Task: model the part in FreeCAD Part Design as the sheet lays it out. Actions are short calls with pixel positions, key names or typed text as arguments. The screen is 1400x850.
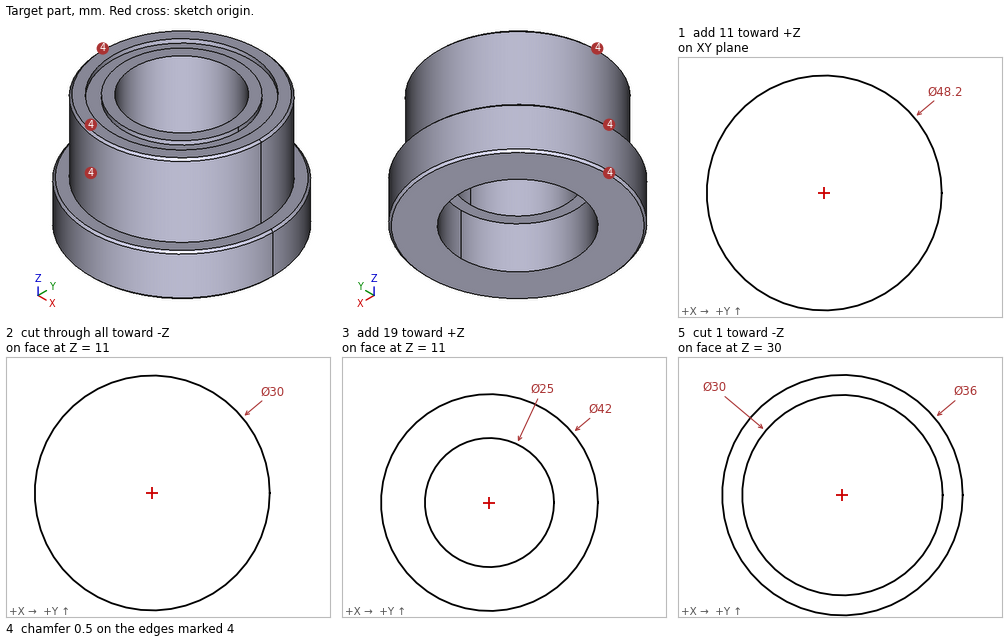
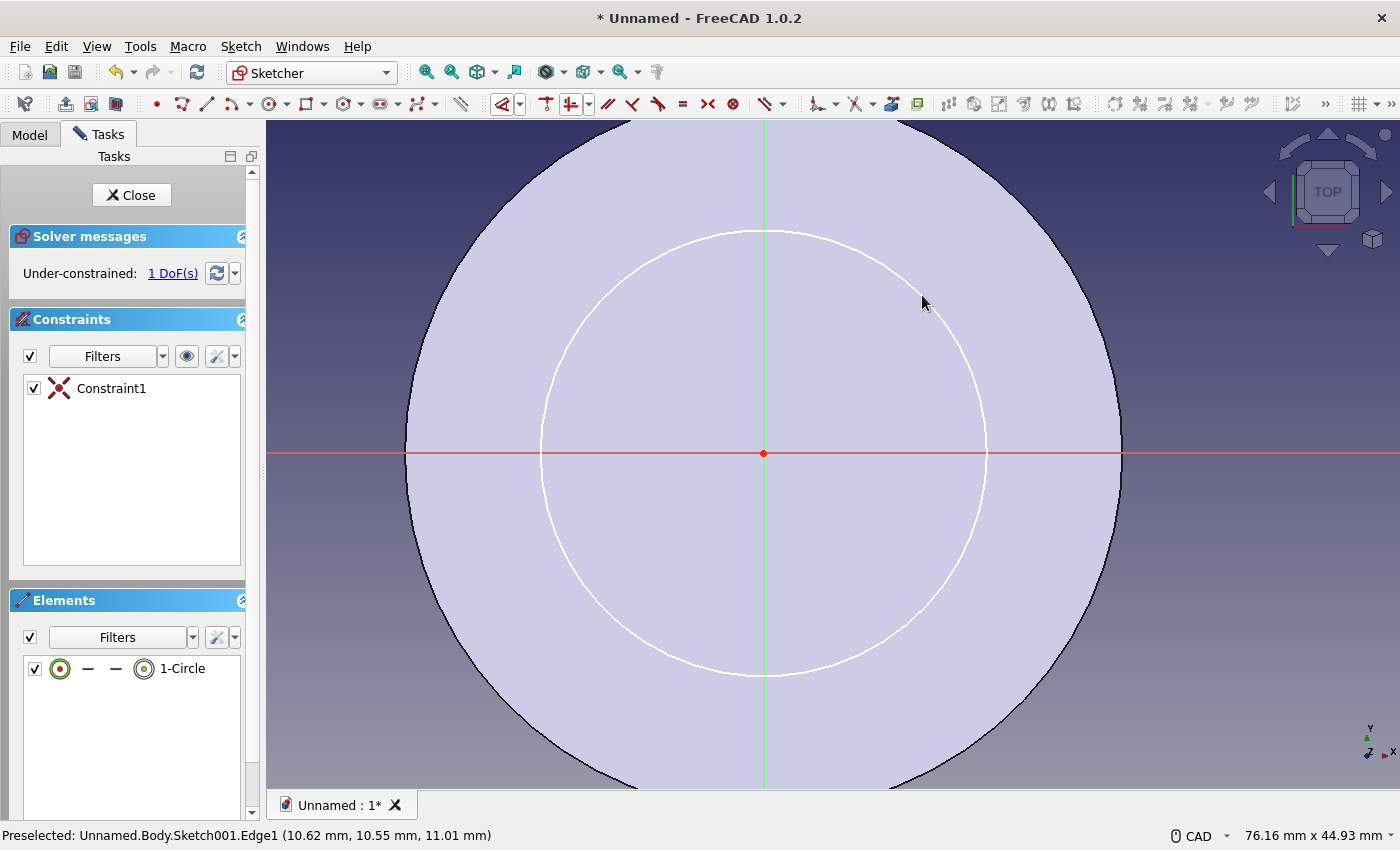
click(502, 104)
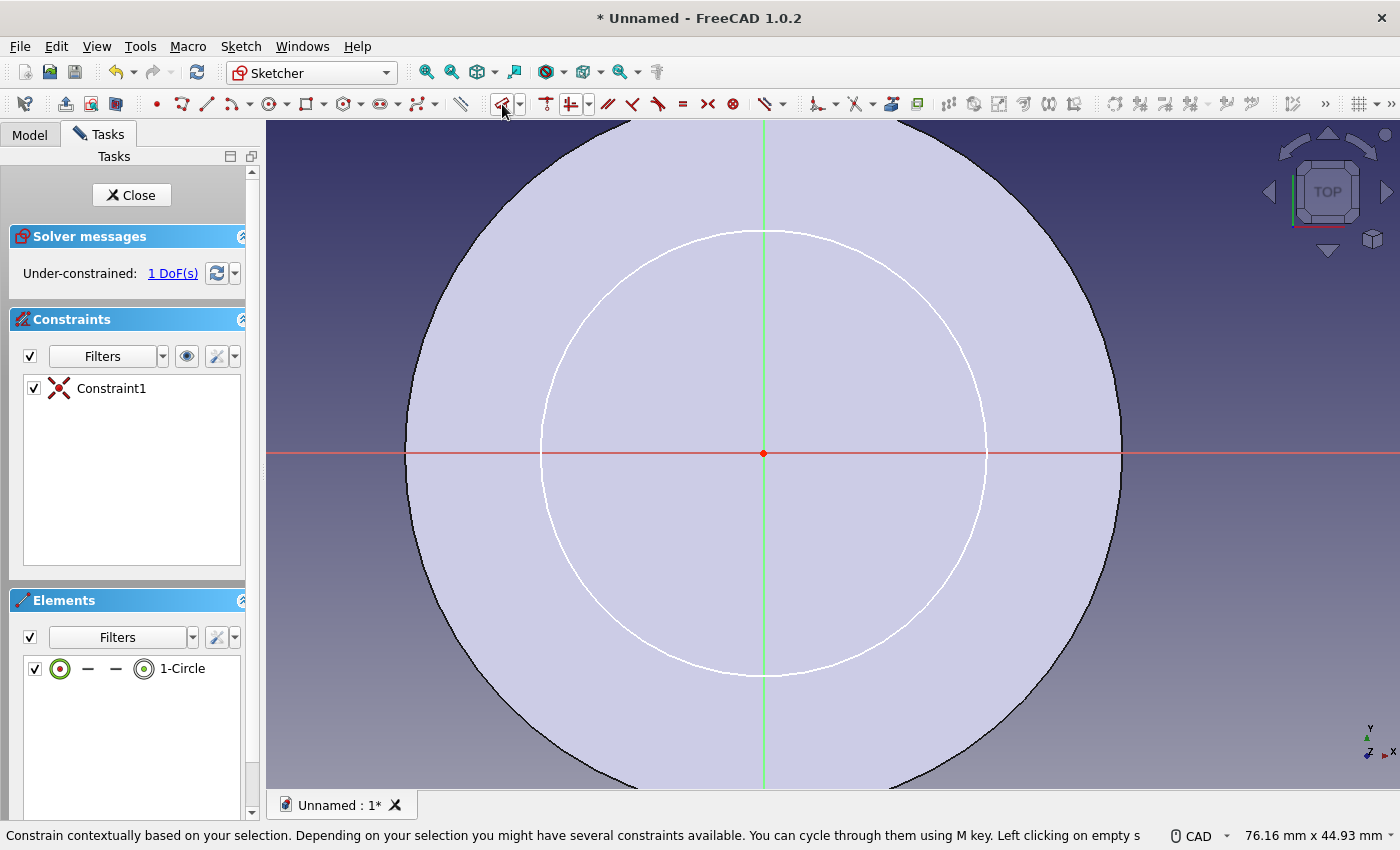
click(921, 295)
click(944, 272)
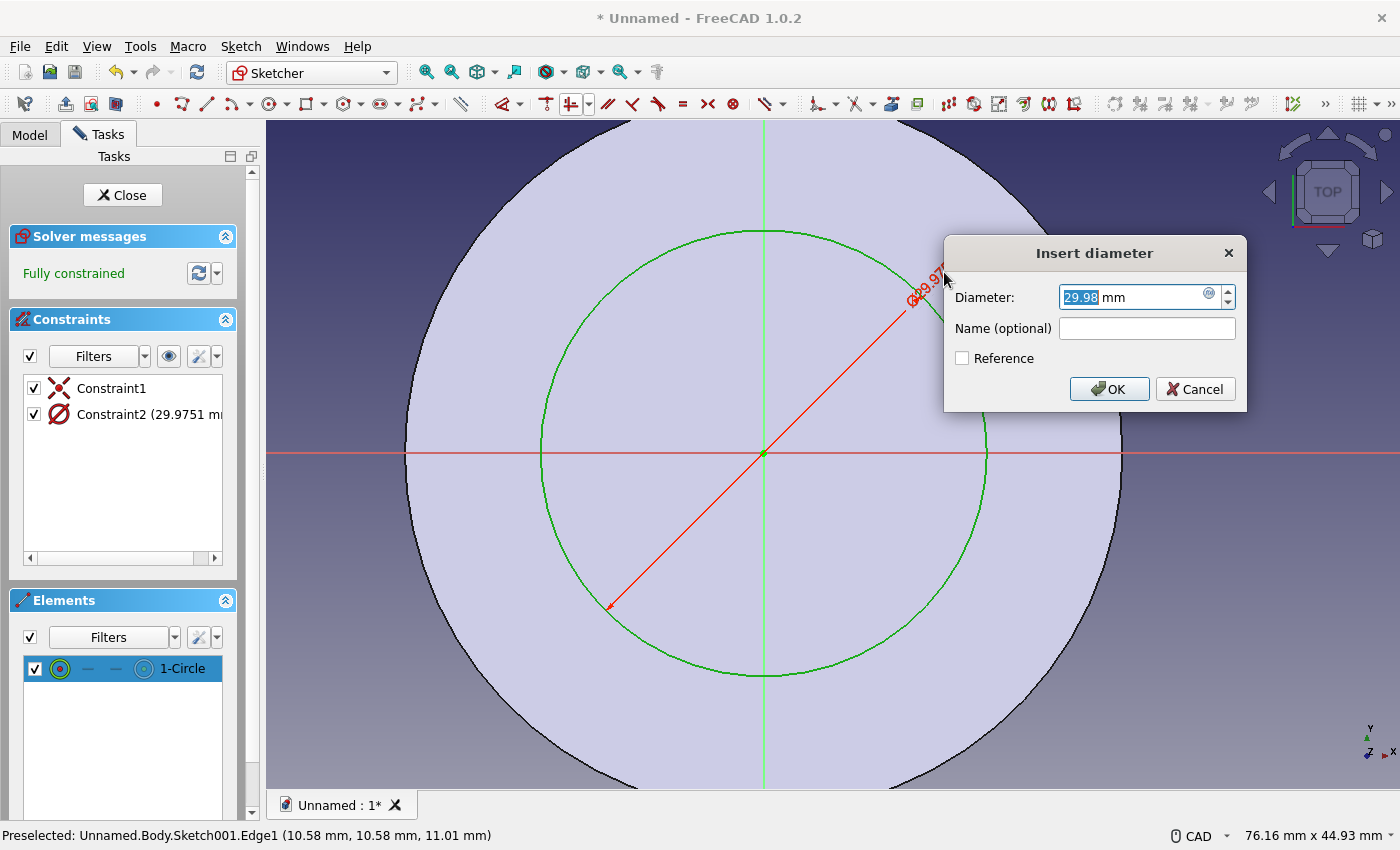
text(30)
key(Return)
key(Escape)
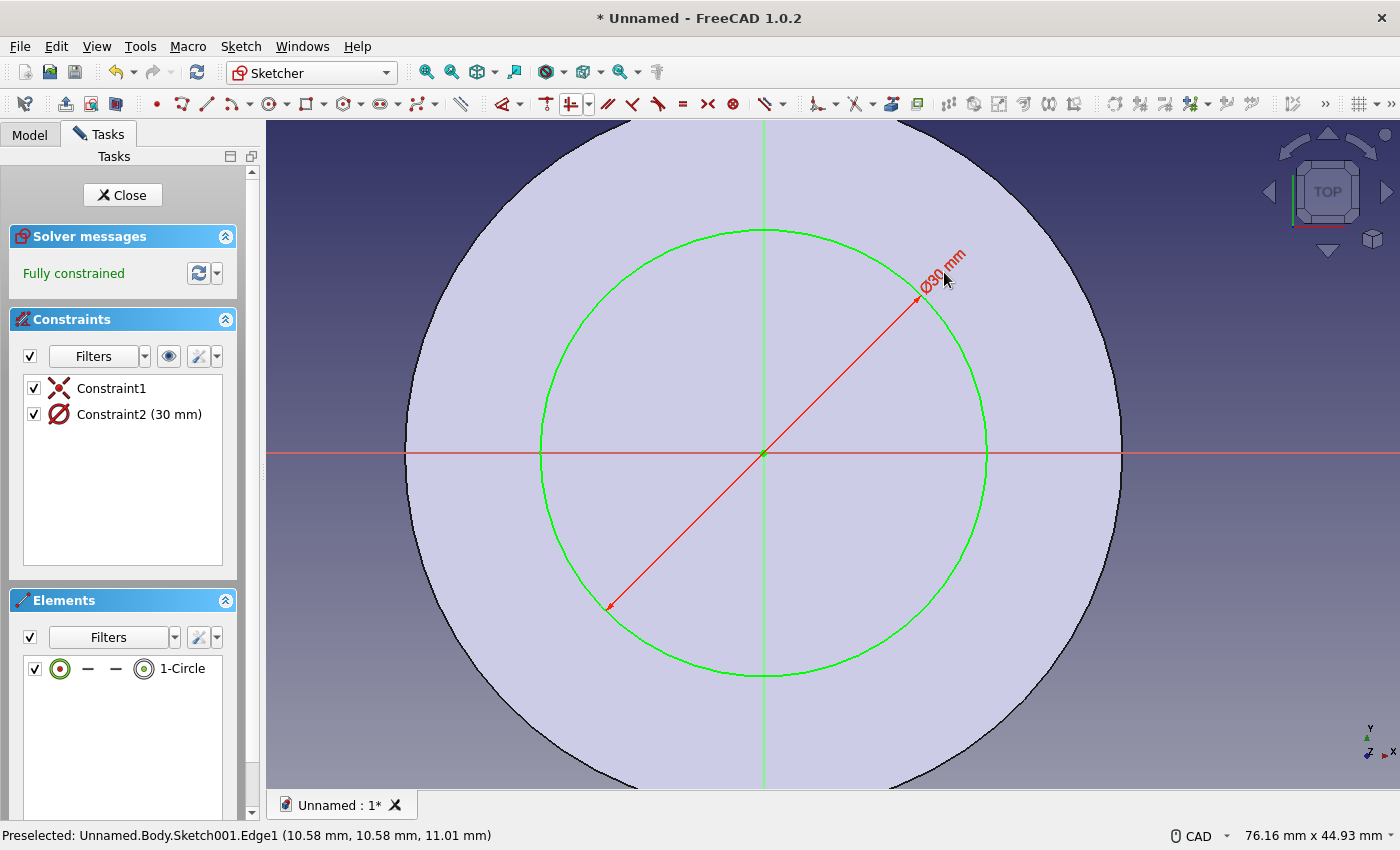
click(123, 195)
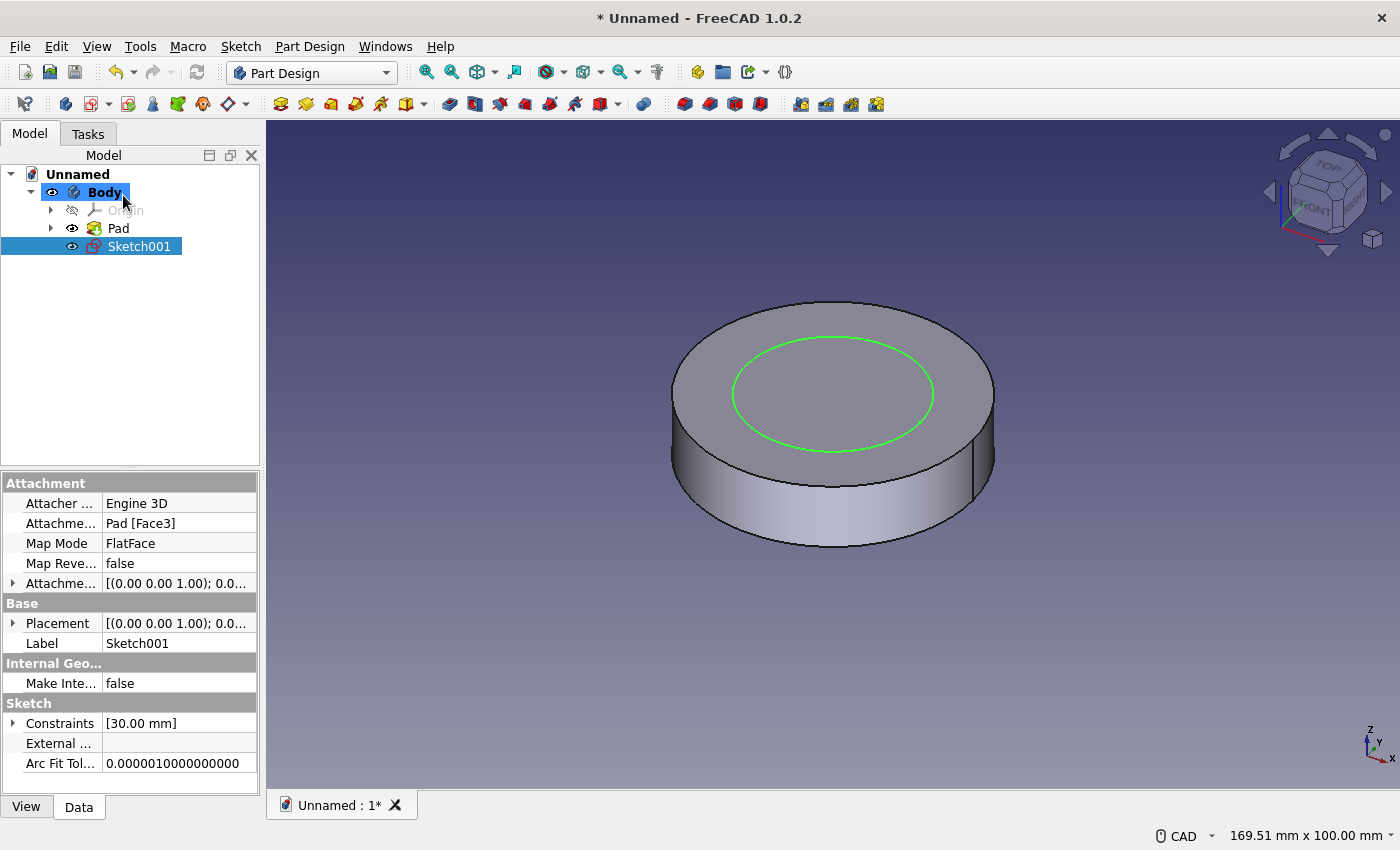
click(450, 104)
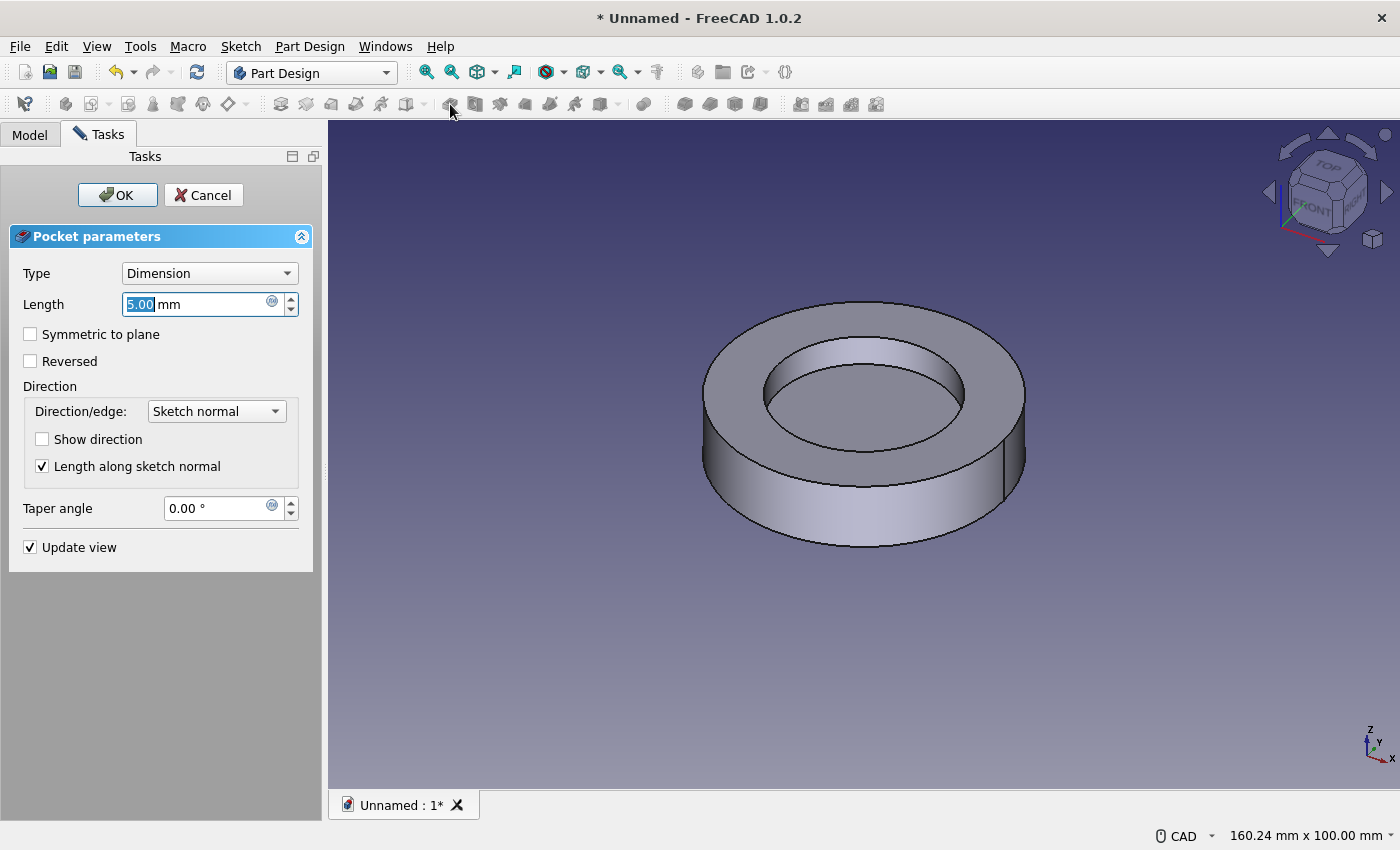
click(210, 274)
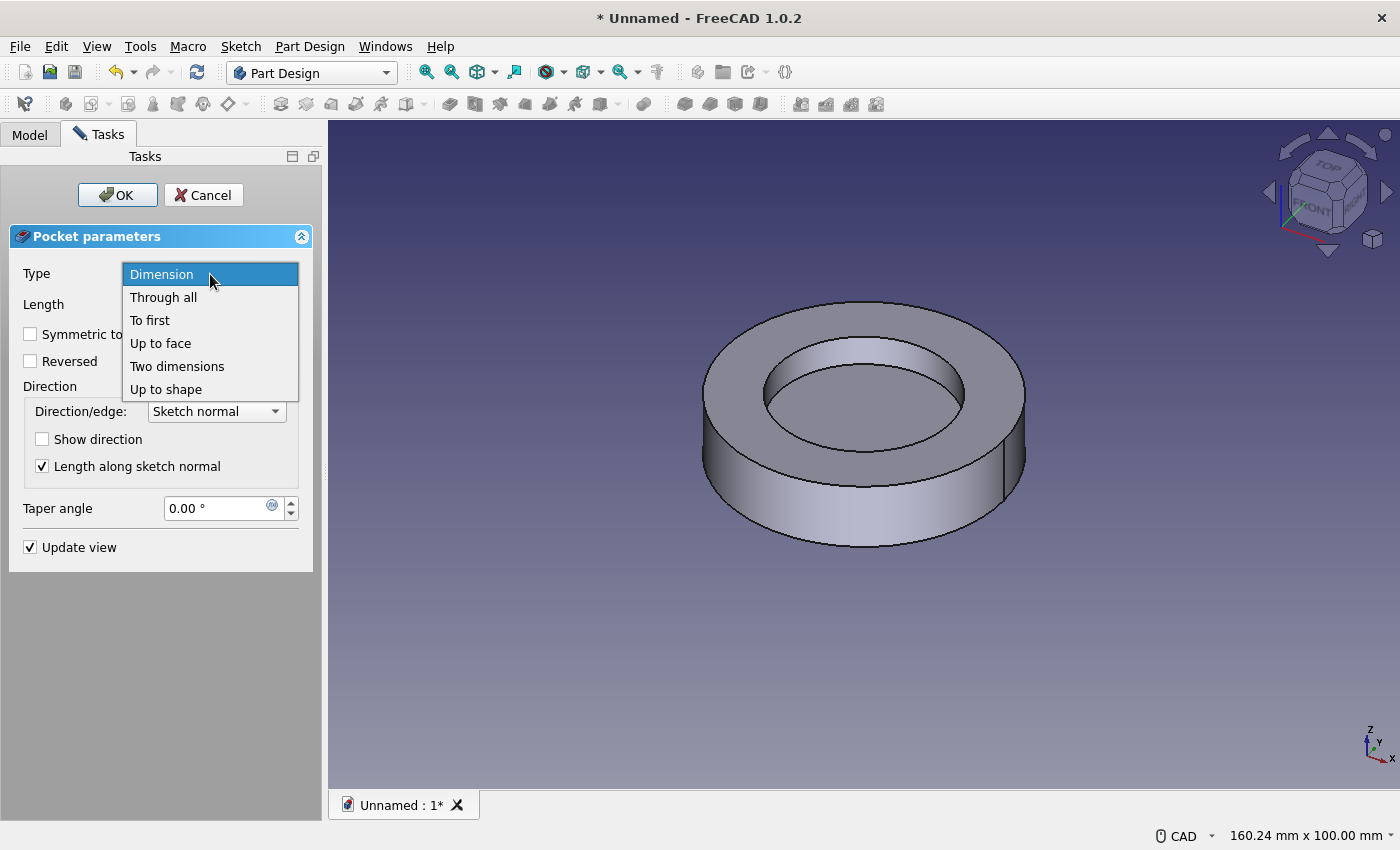
click(208, 298)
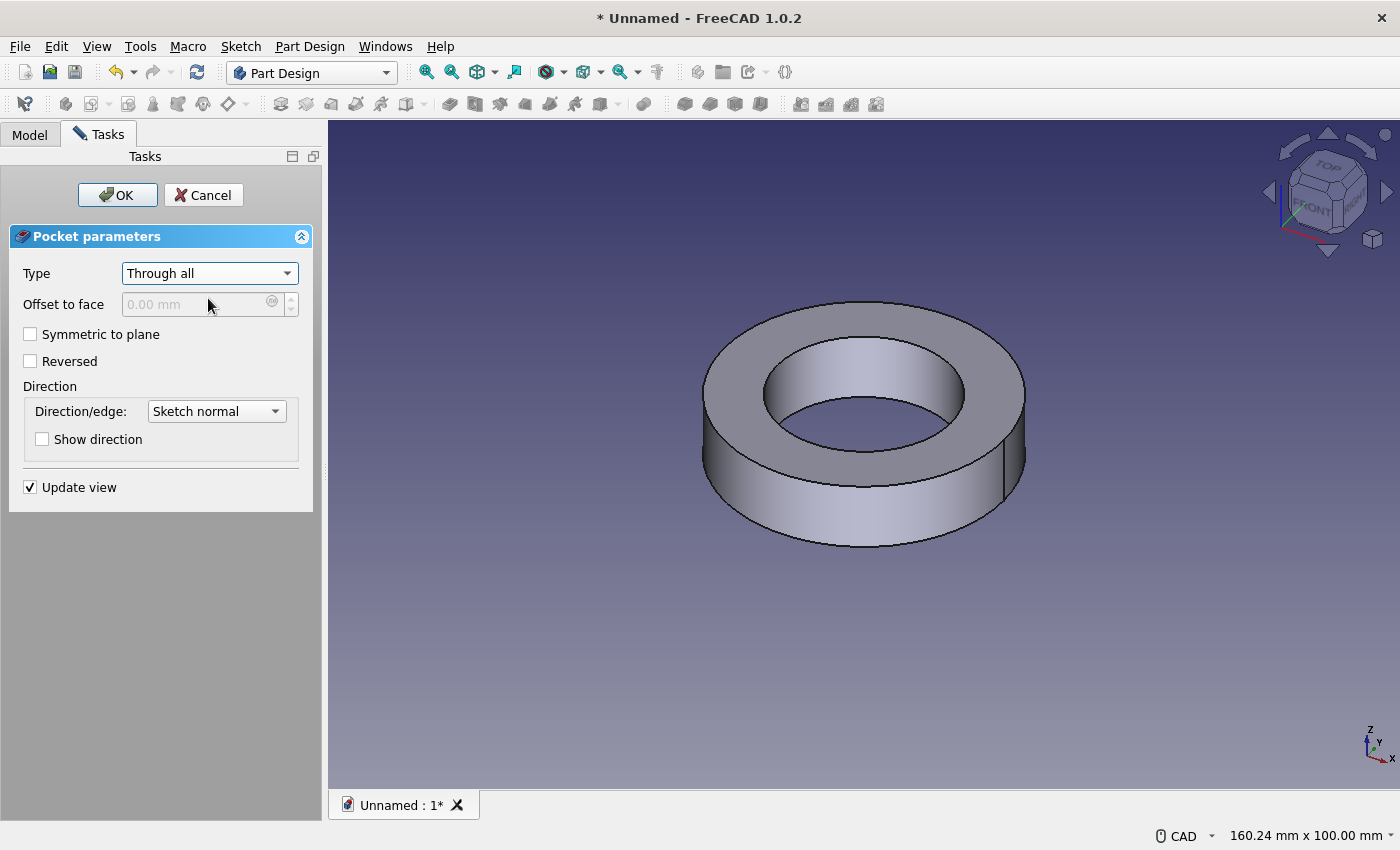
click(118, 195)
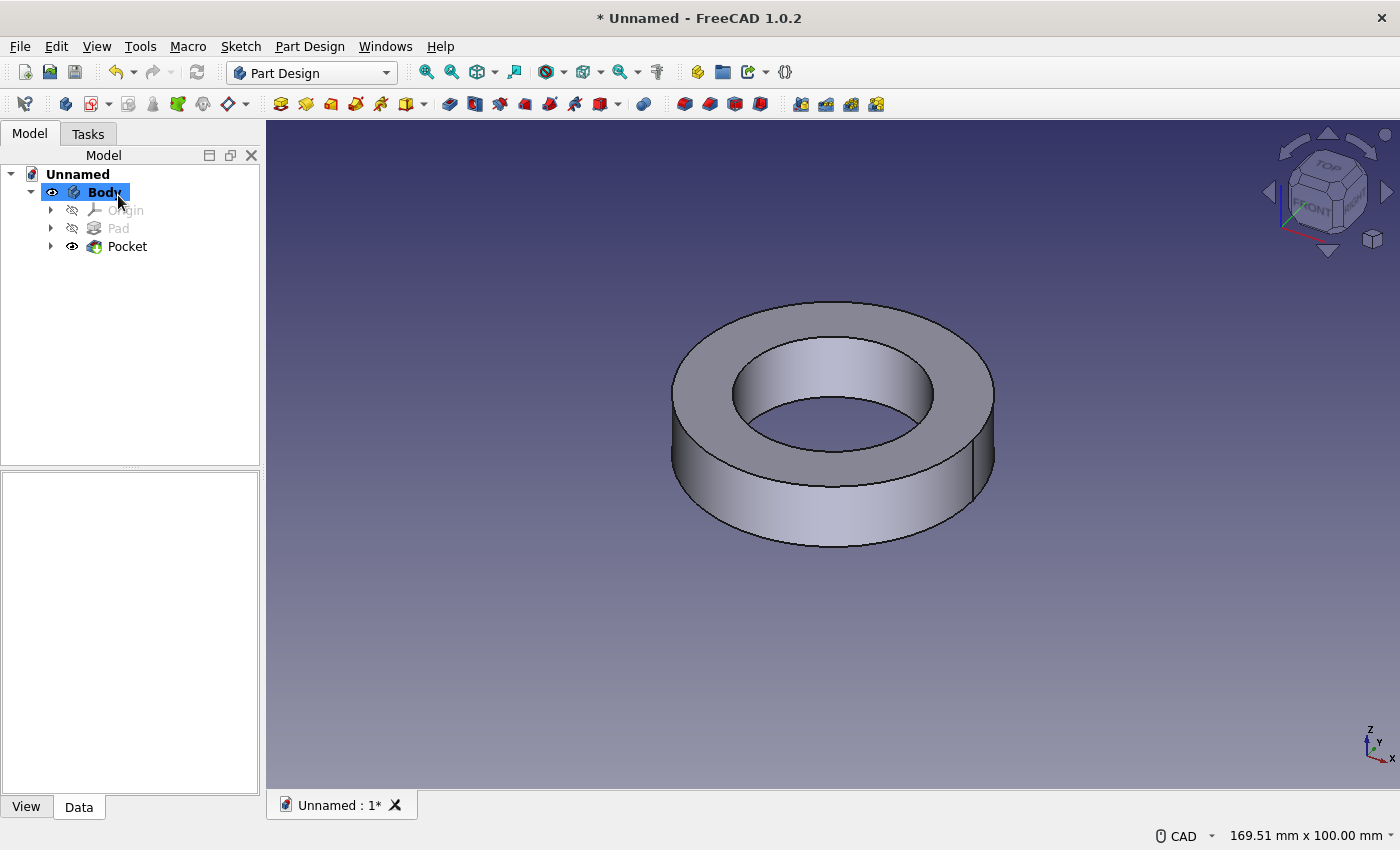
click(867, 465)